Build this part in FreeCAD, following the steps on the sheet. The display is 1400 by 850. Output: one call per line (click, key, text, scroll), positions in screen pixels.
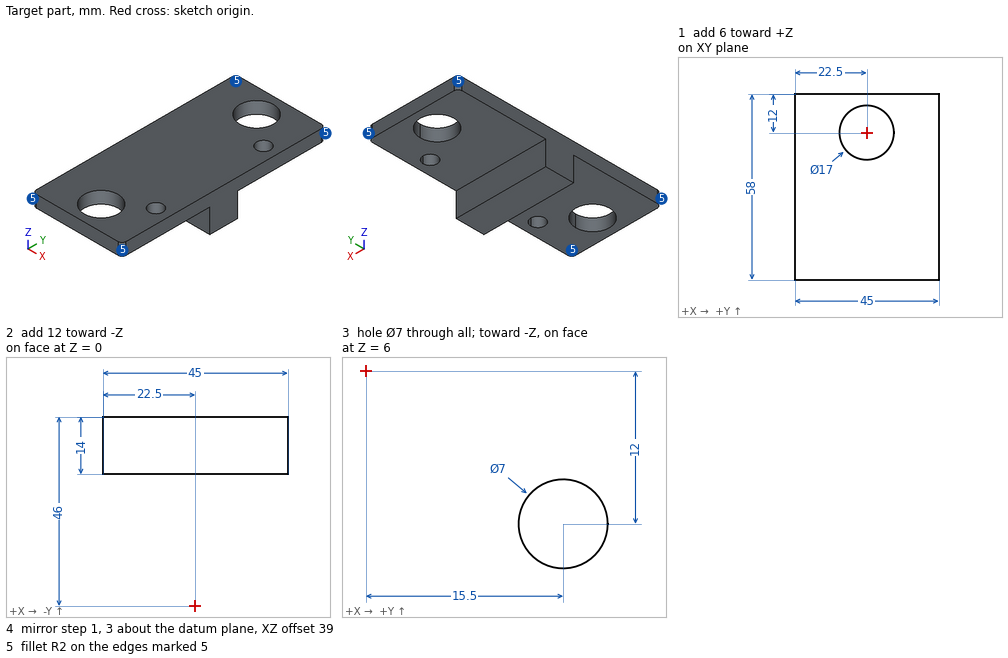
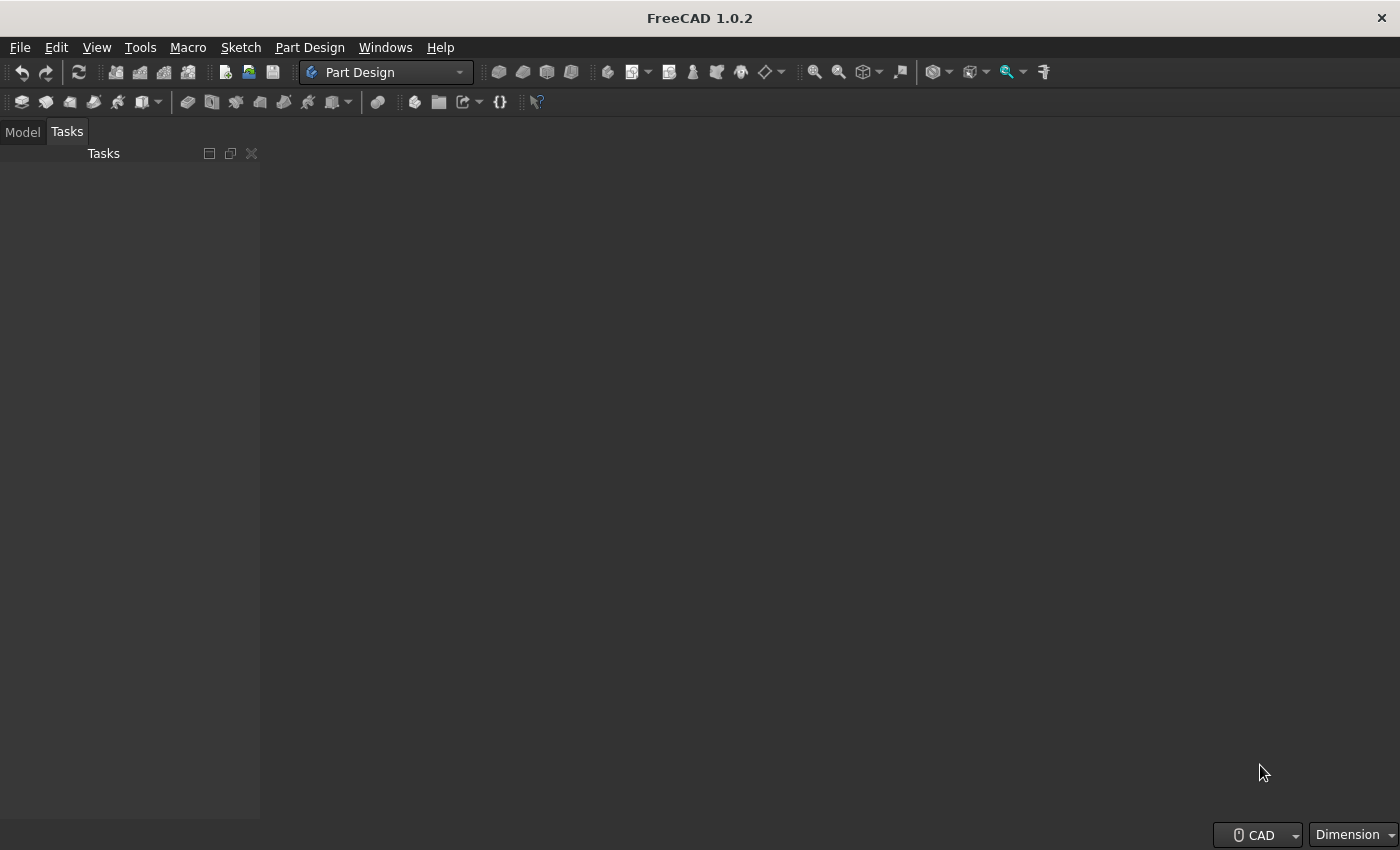
click(226, 72)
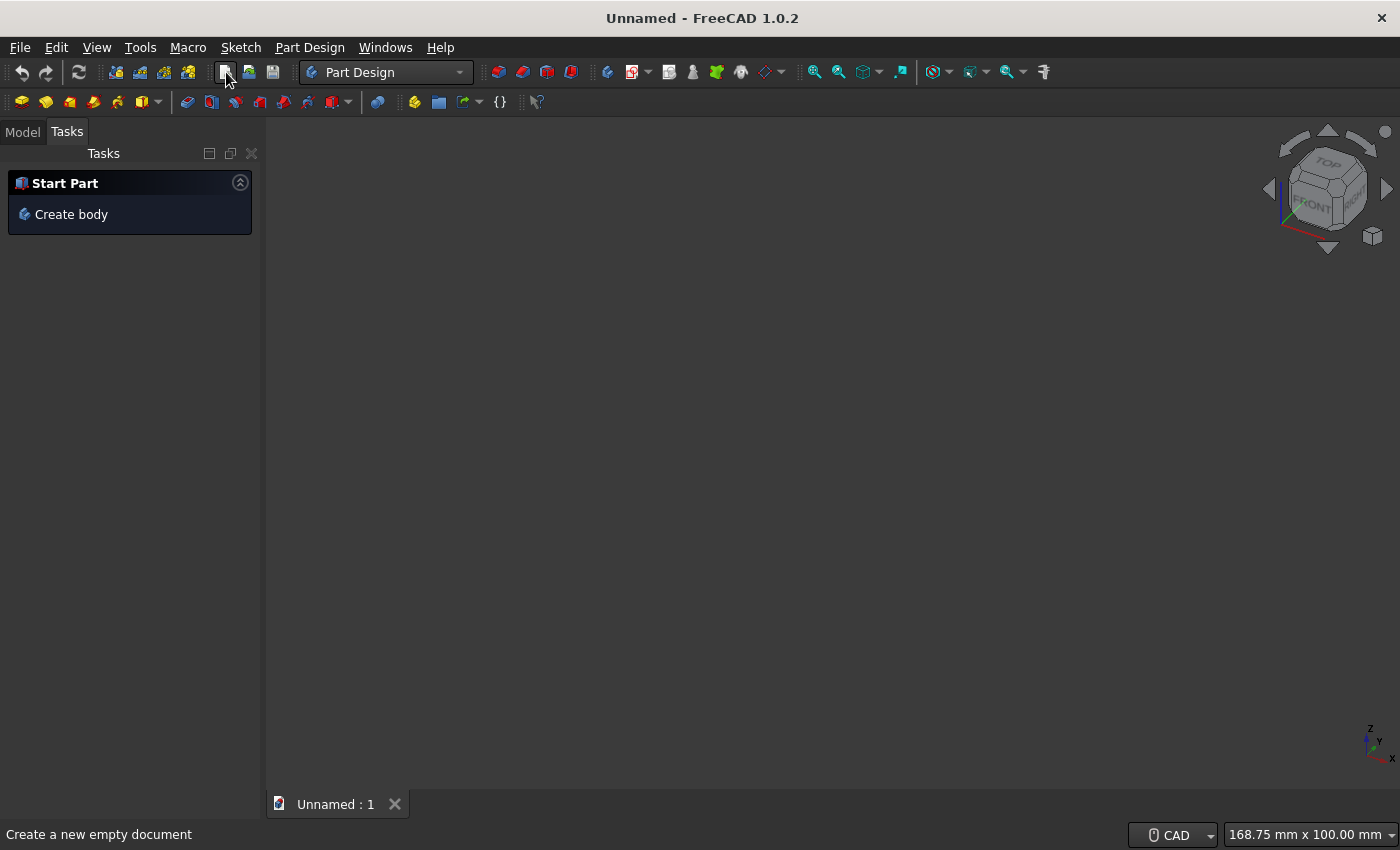
click(632, 72)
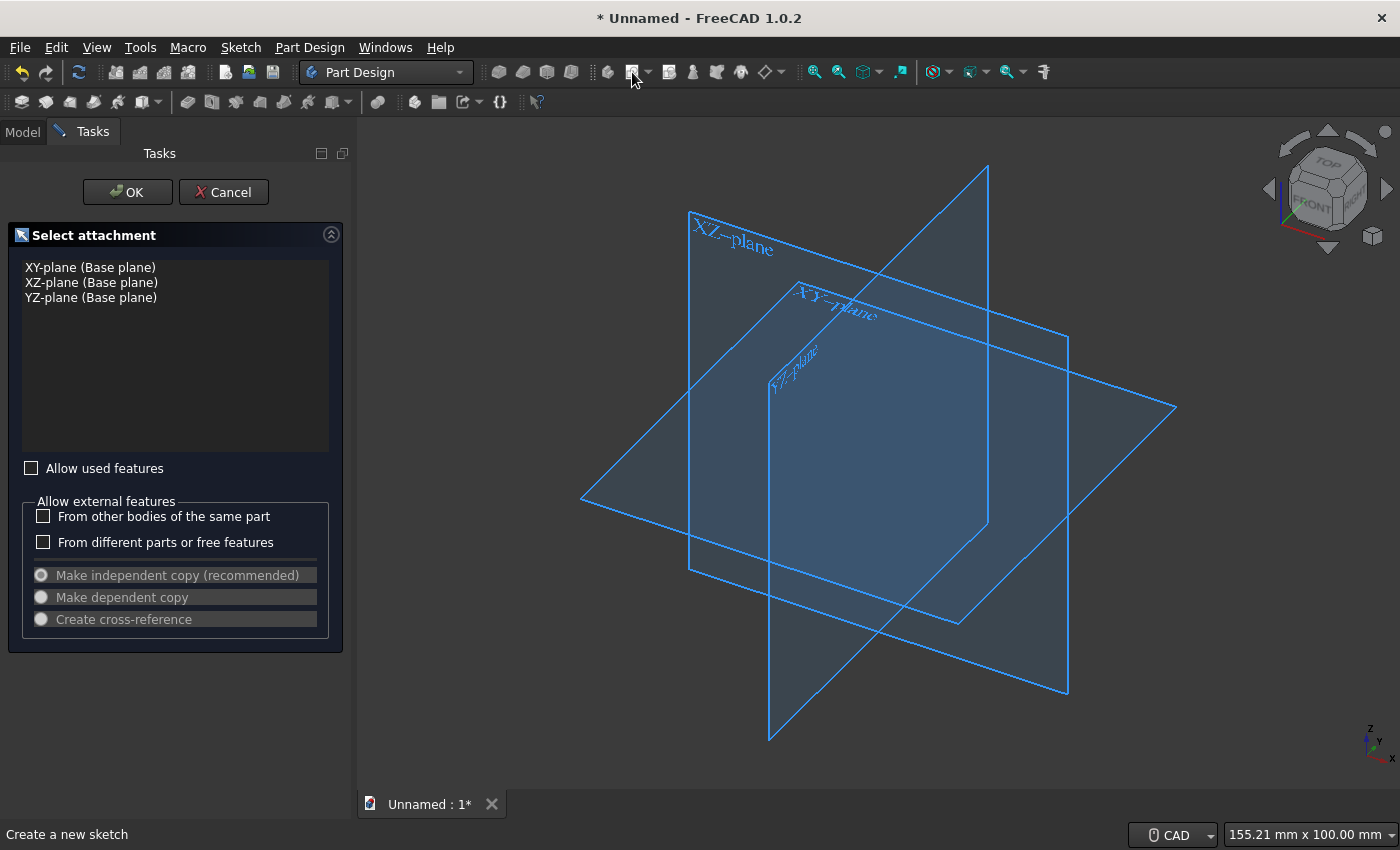
click(82, 268)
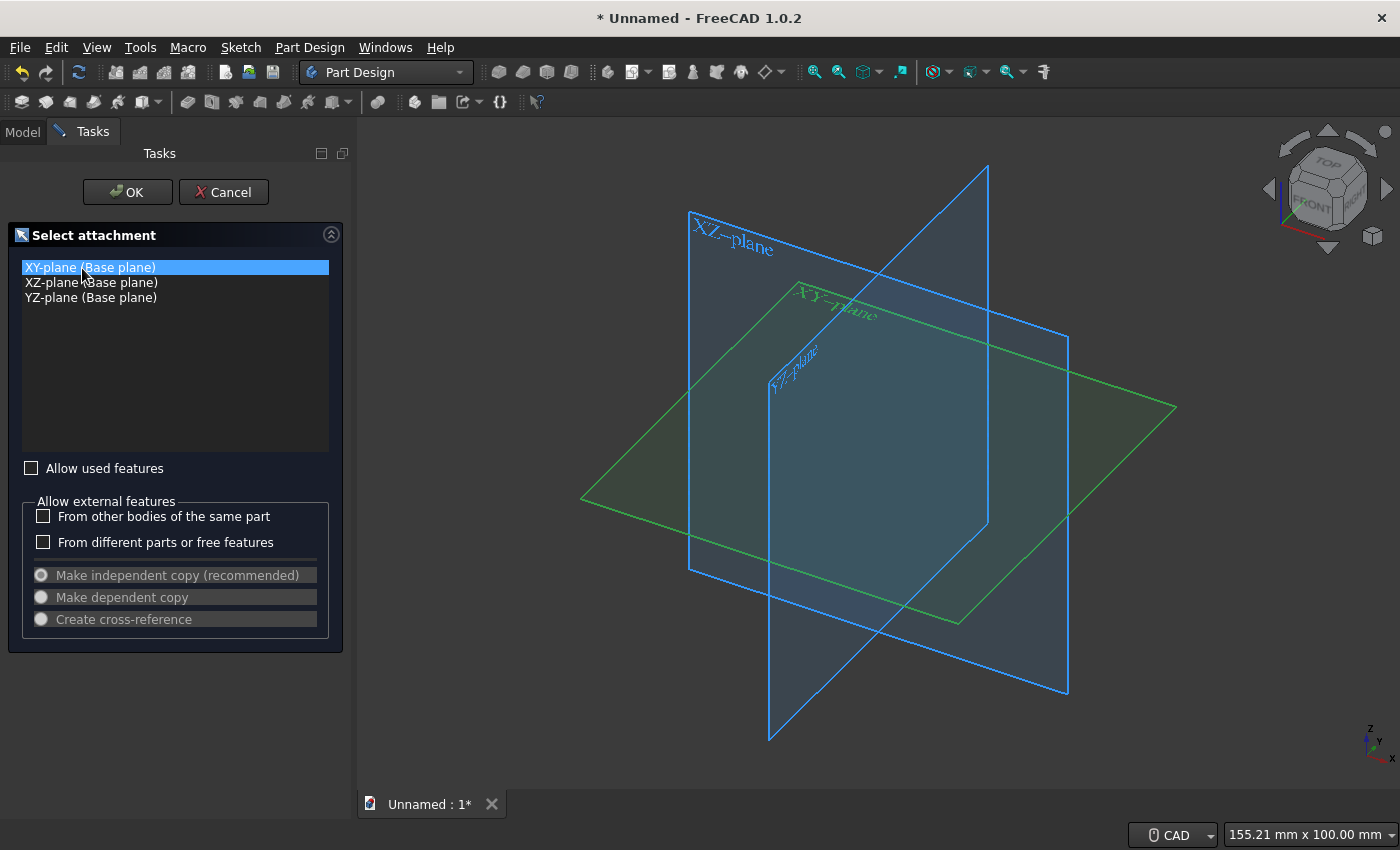
click(128, 192)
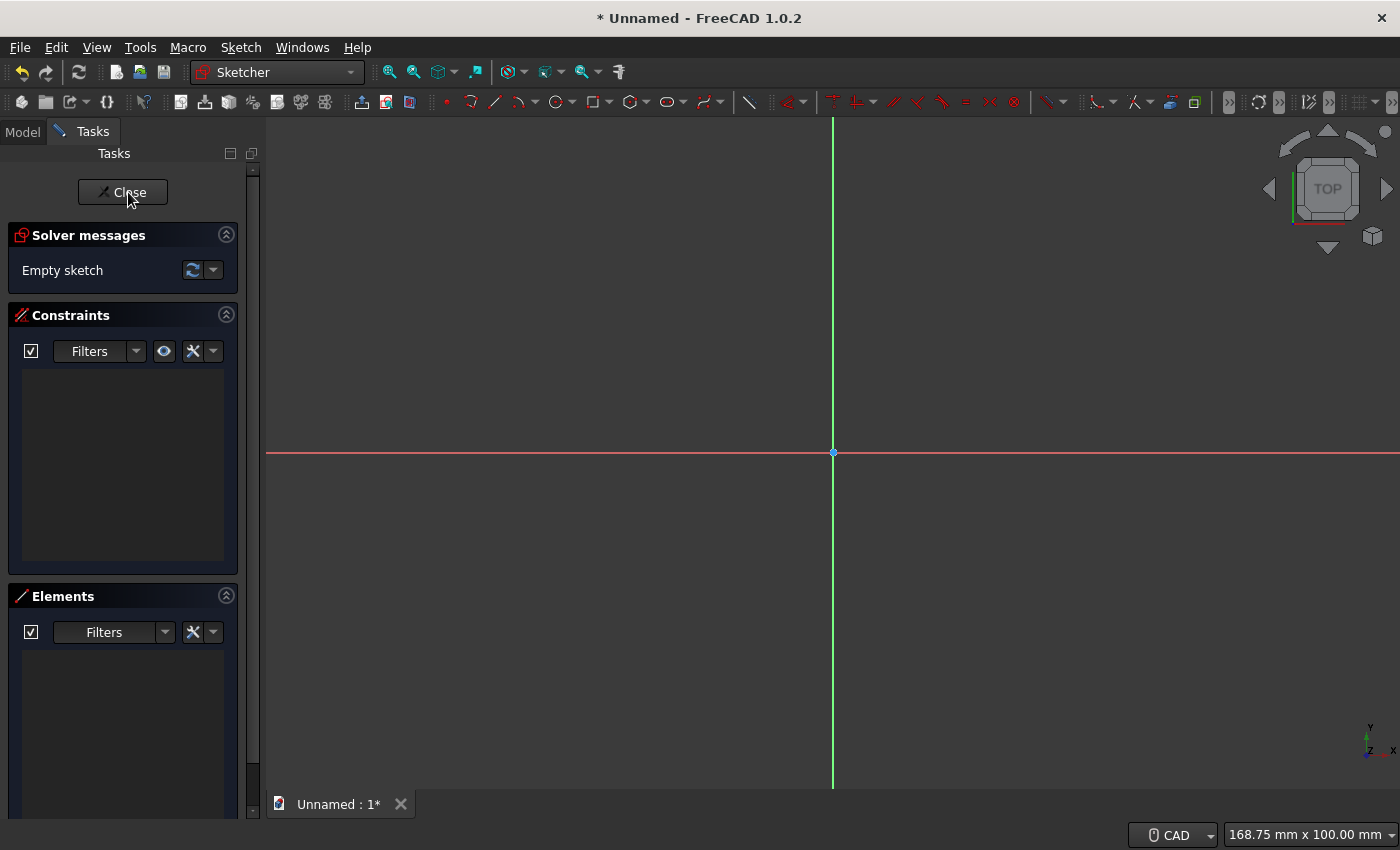
scroll(455, 145, down, 1)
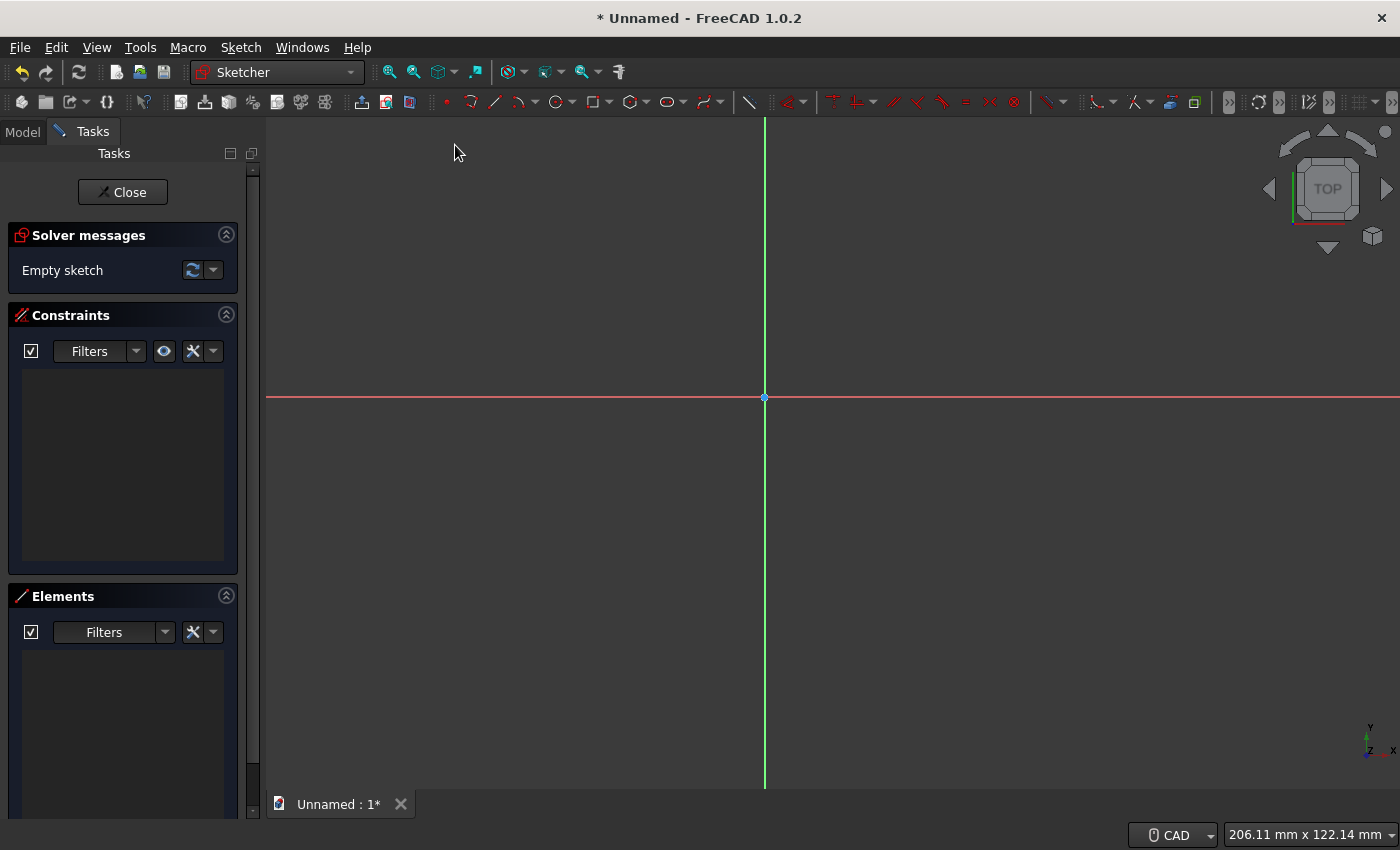
scroll(765, 567, up, 2)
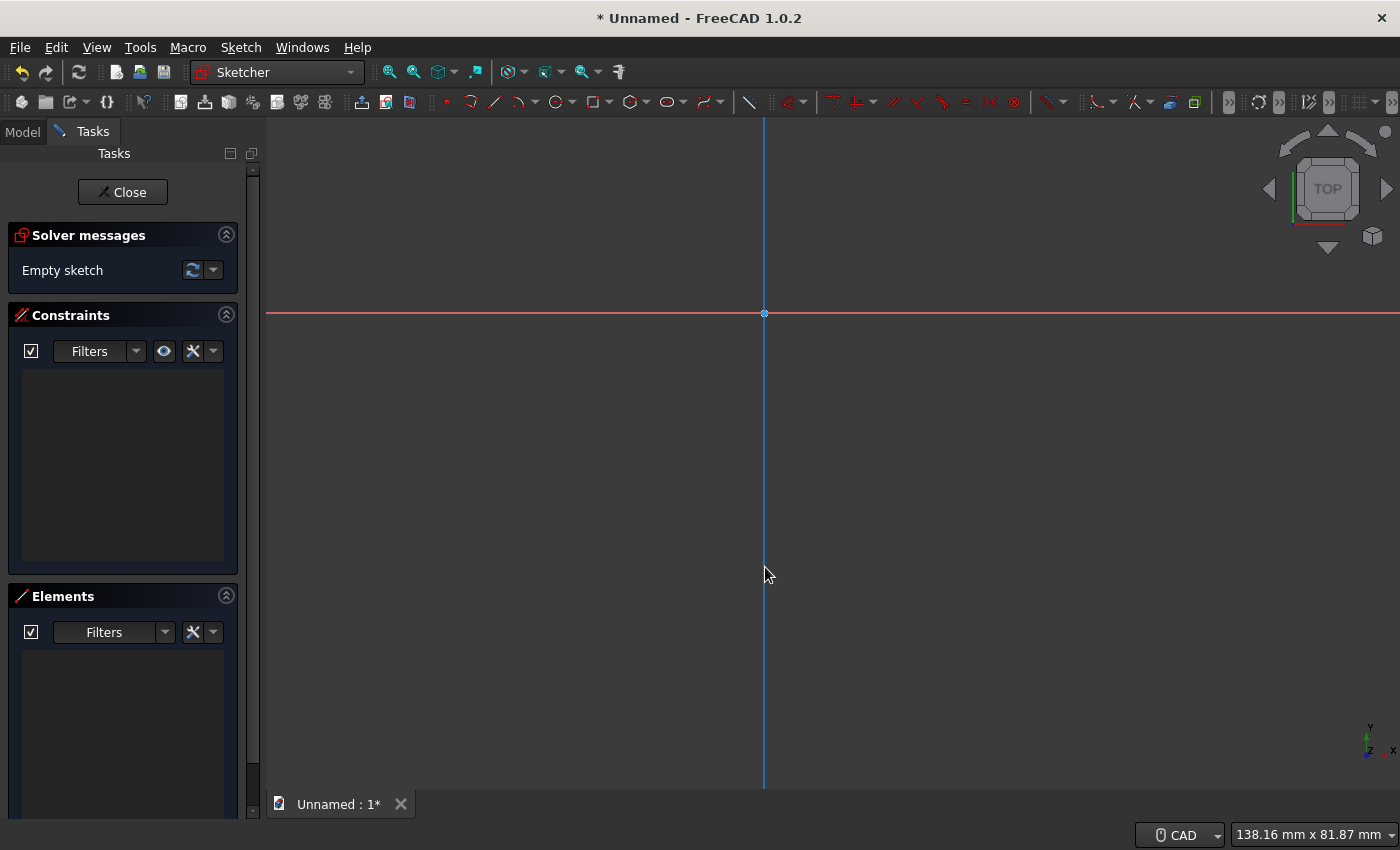
click(594, 102)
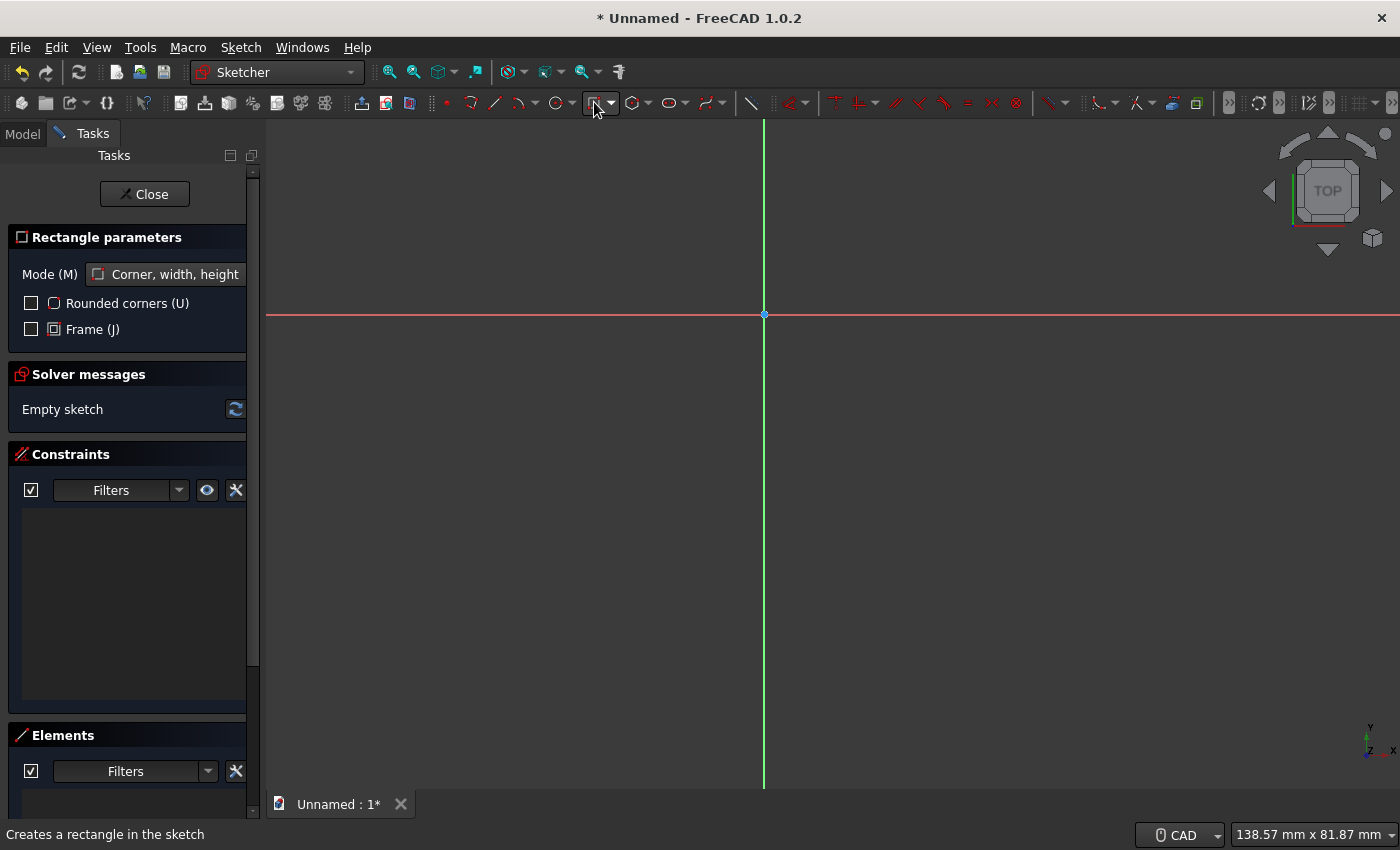
click(580, 217)
click(948, 691)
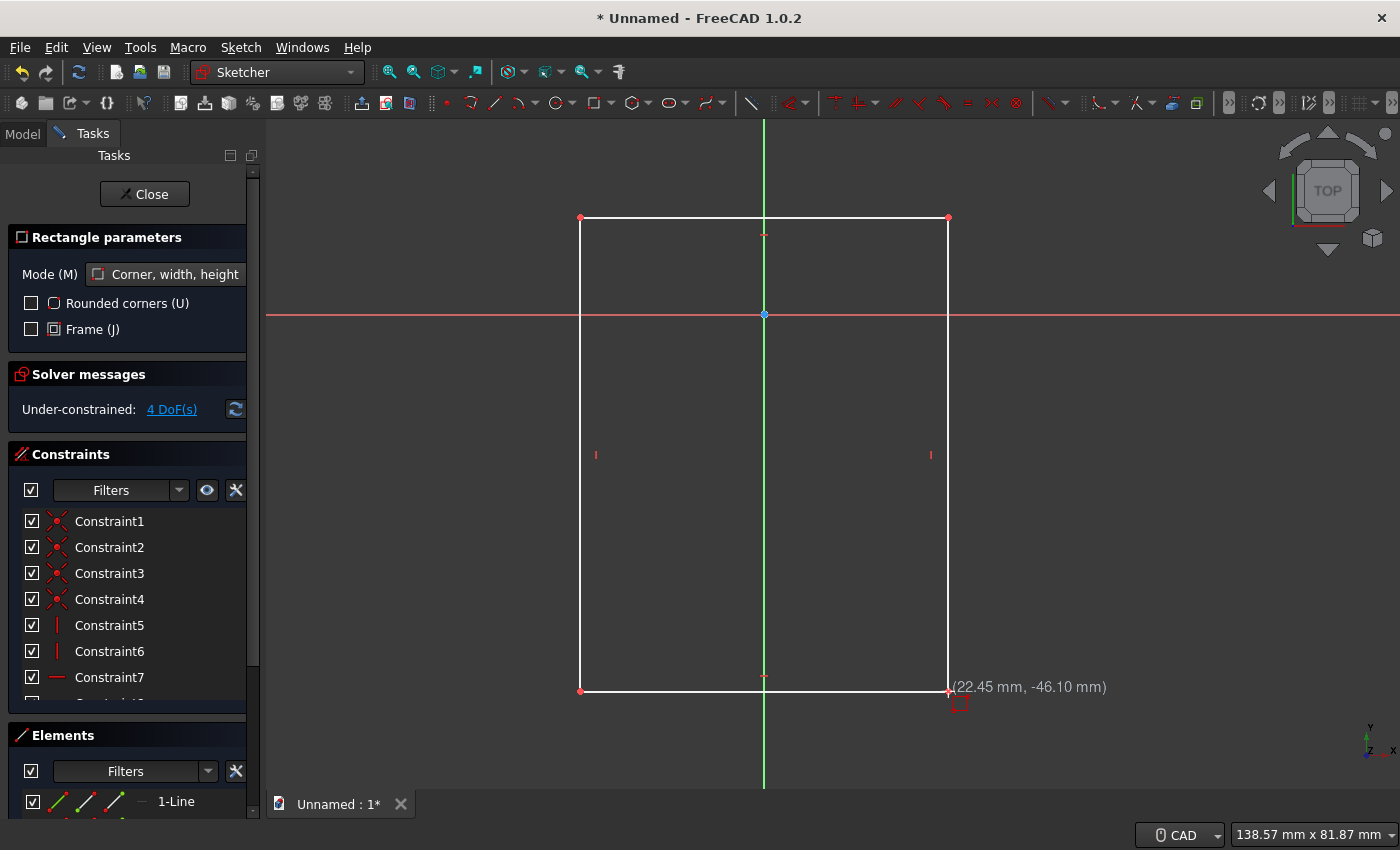
click(556, 104)